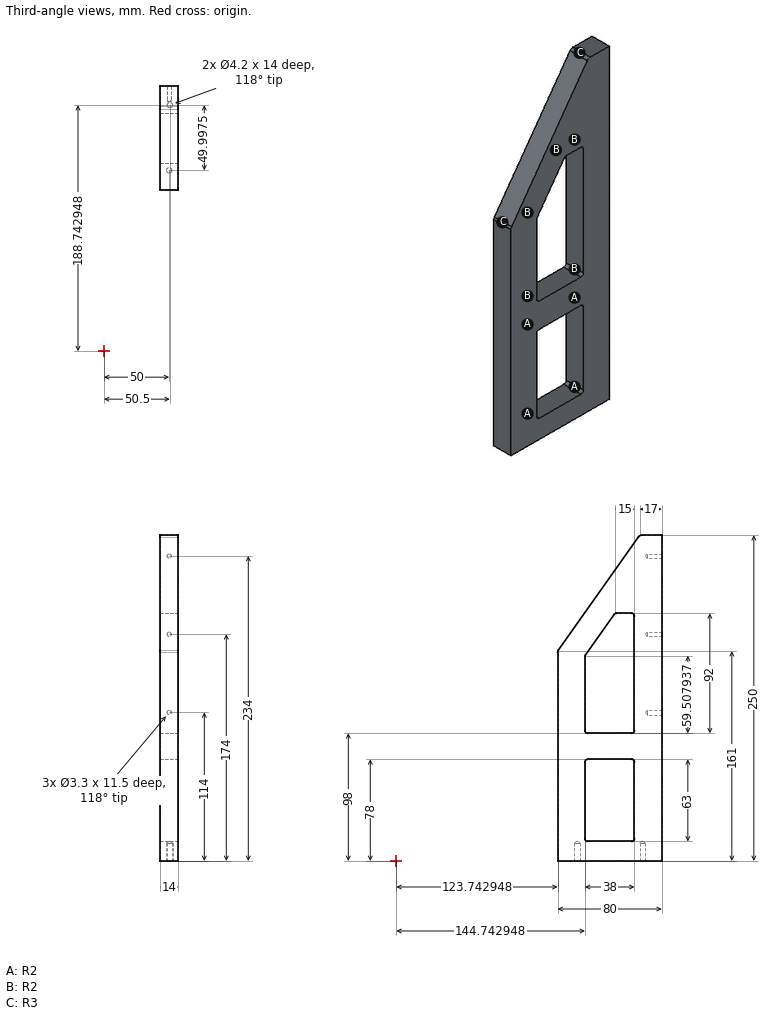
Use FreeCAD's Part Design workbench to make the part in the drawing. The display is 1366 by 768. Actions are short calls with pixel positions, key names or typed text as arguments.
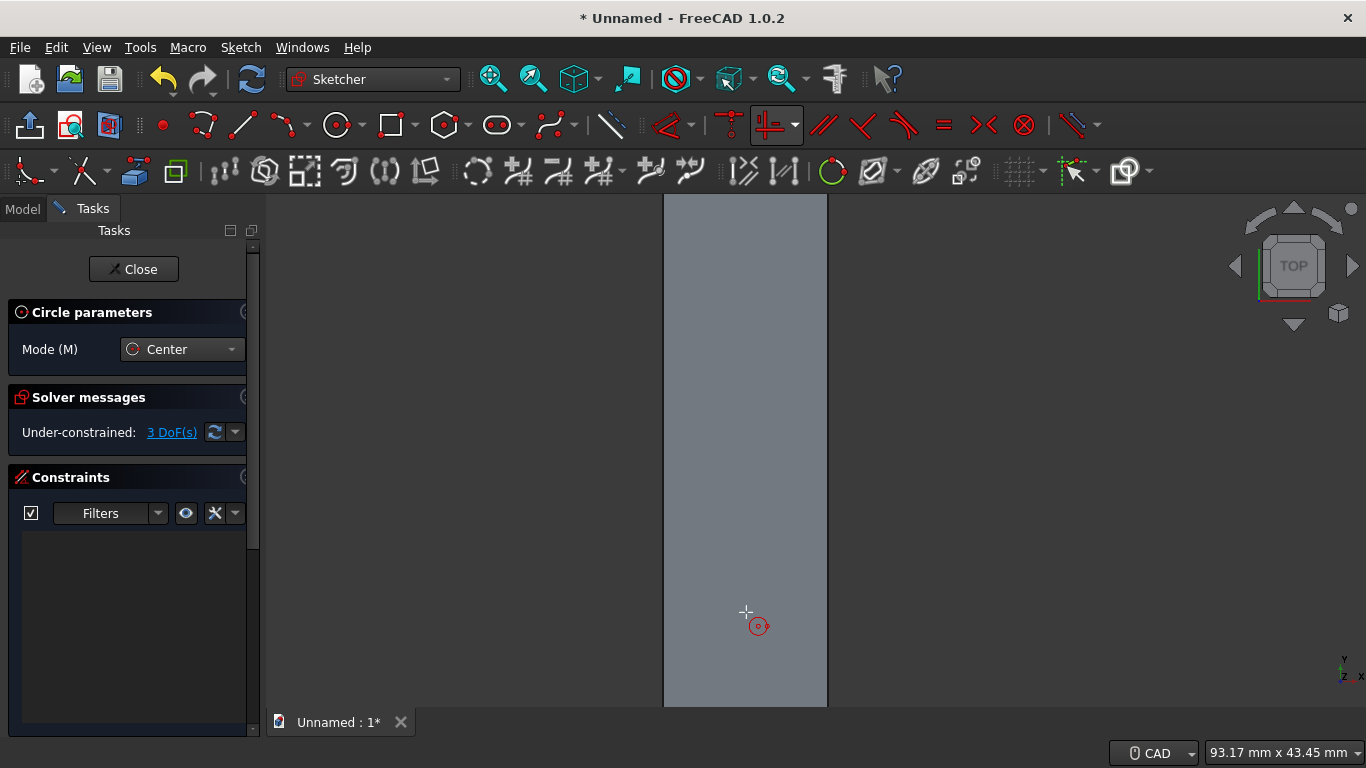
click(746, 612)
click(763, 595)
key(Escape)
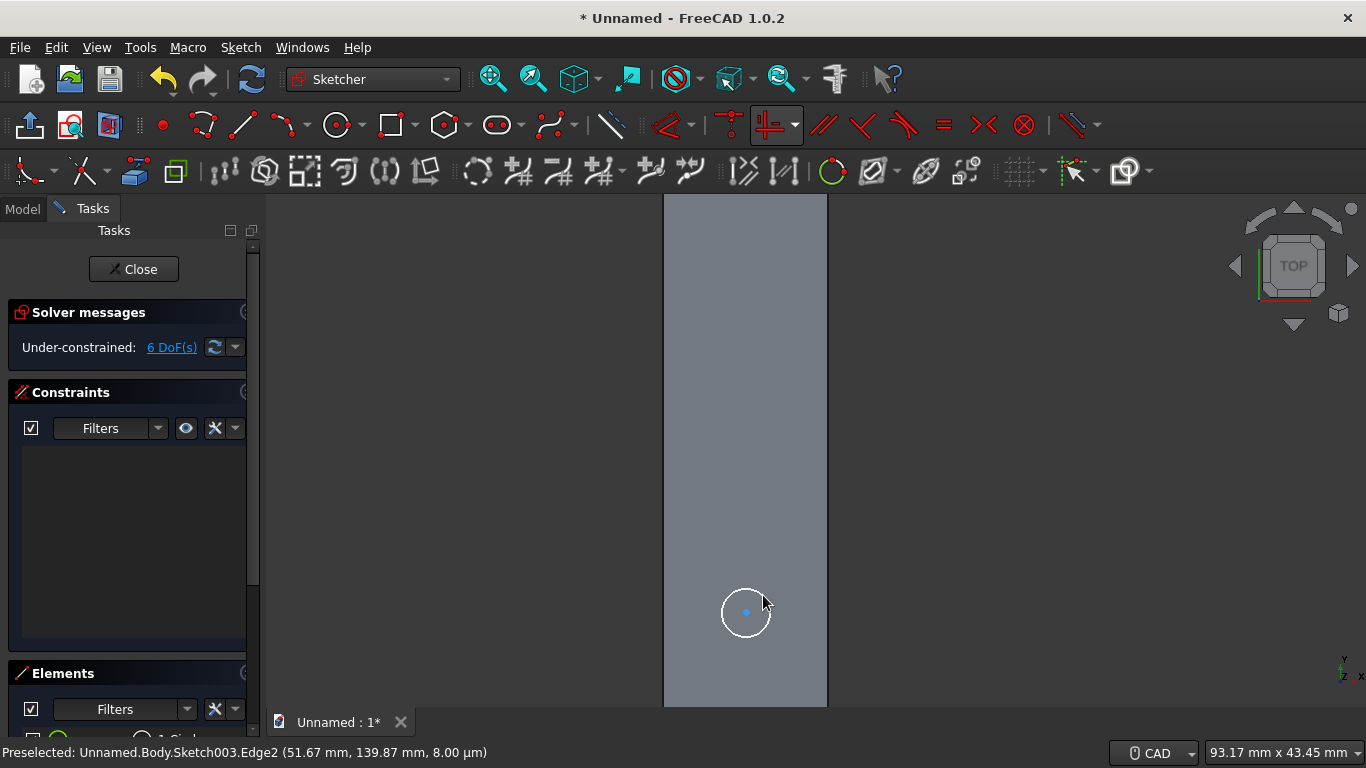
scroll(746, 613, down, 3)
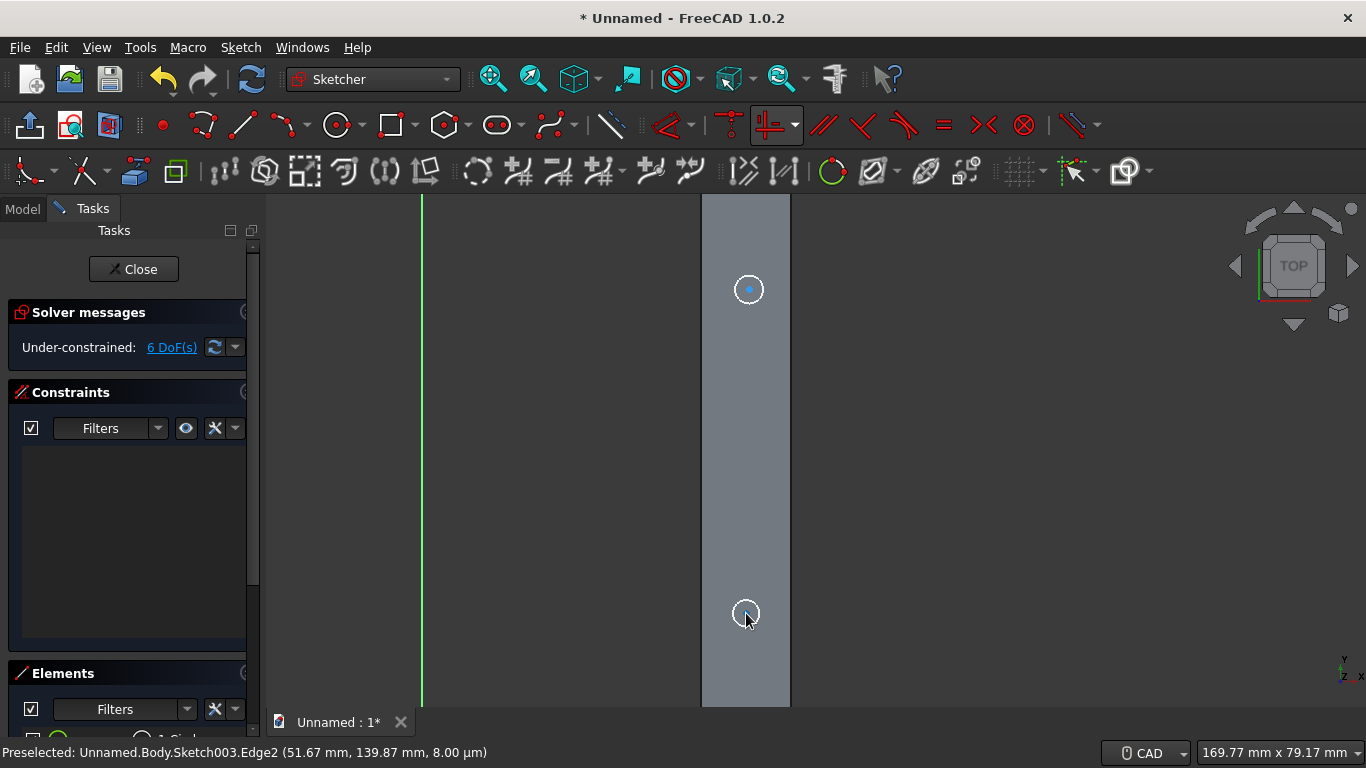
click(759, 280)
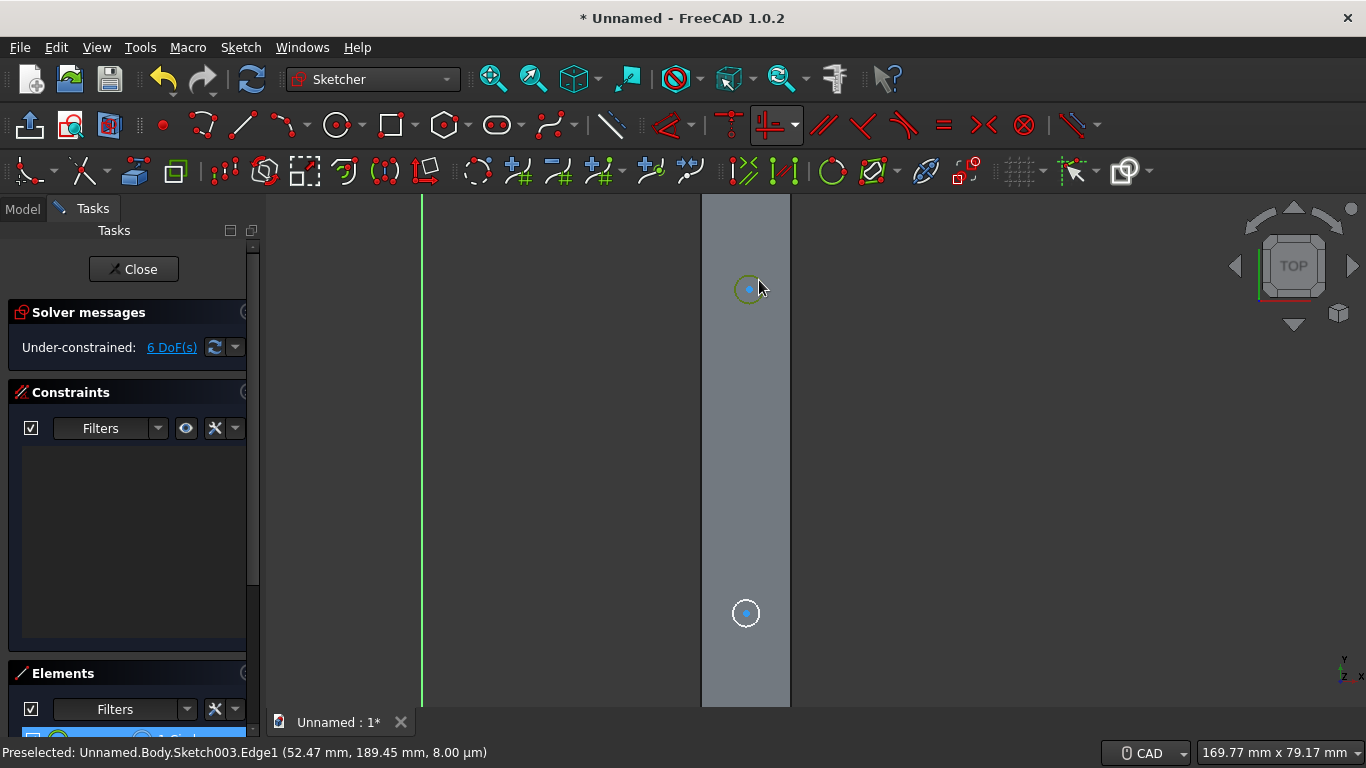
click(755, 604)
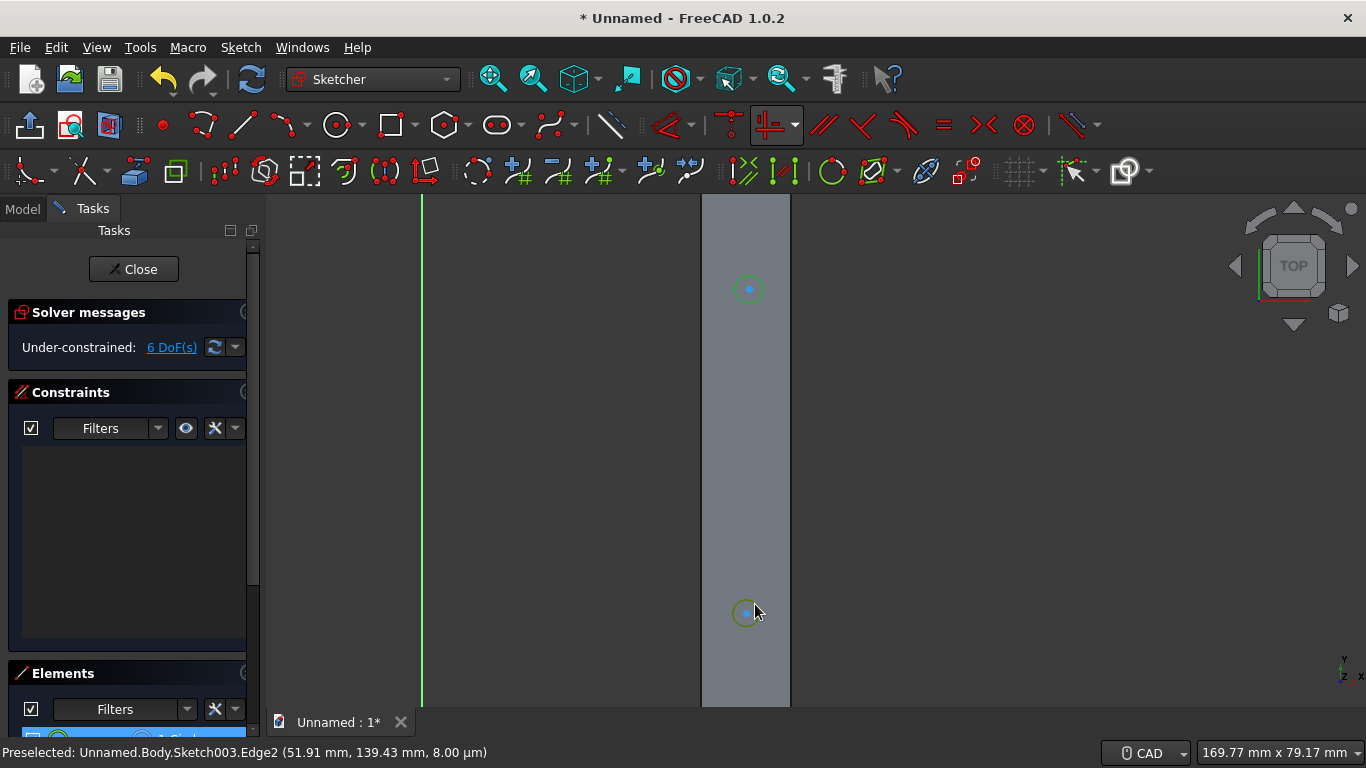
click(944, 126)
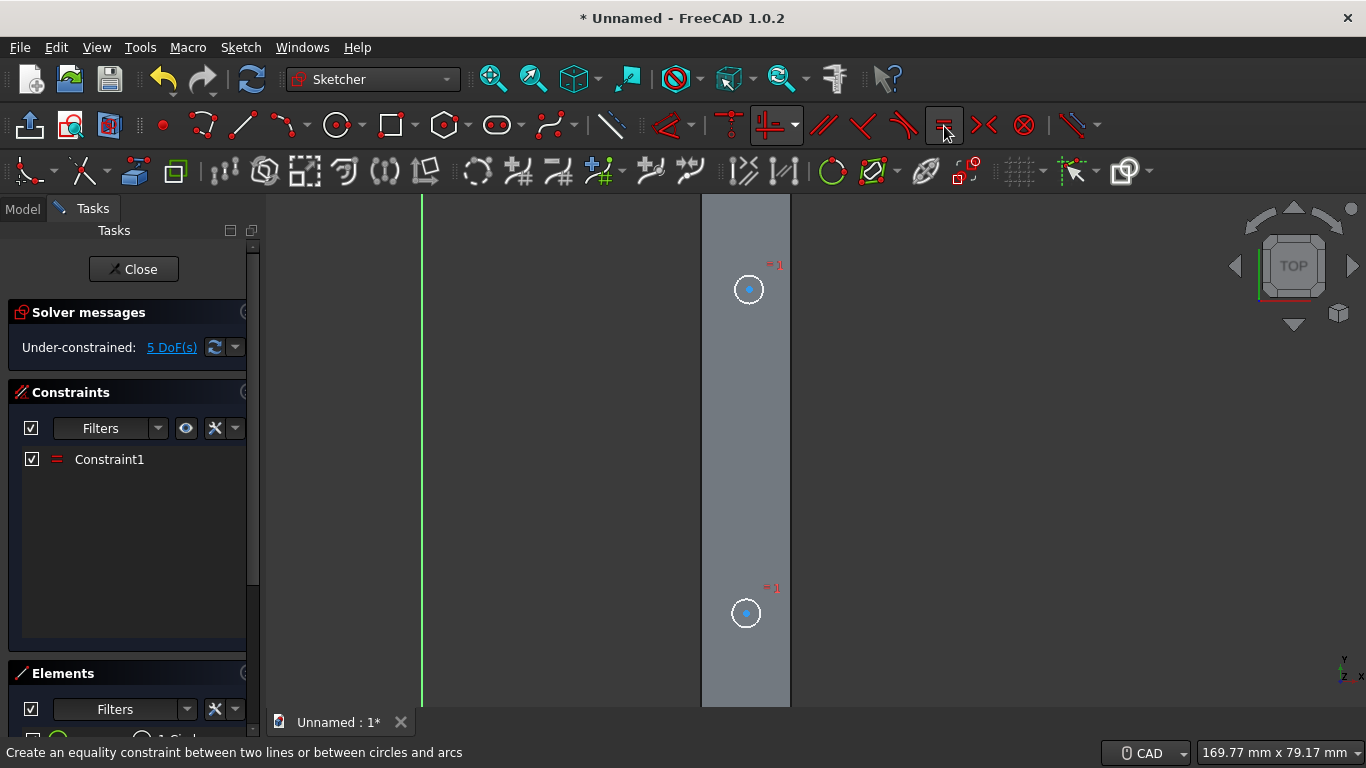
click(666, 126)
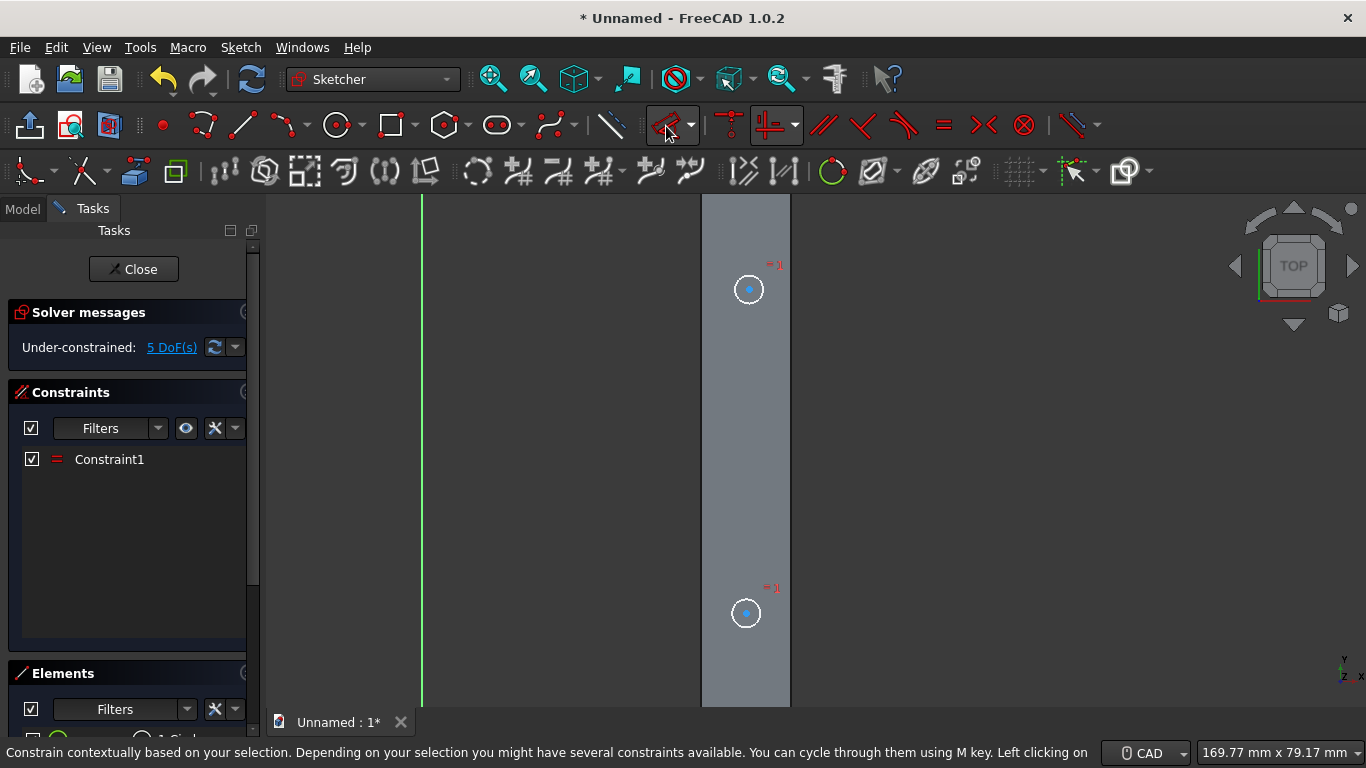
scroll(759, 280, up, 2)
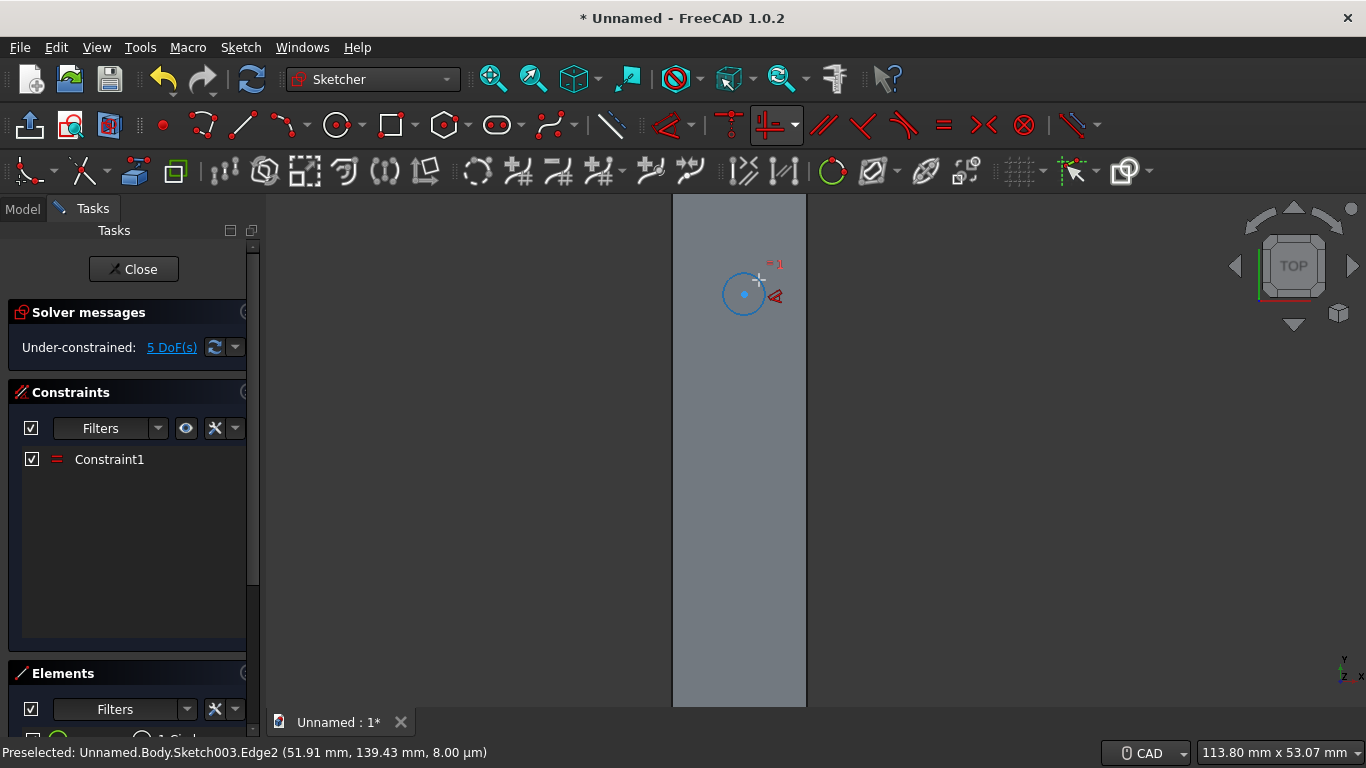
click(759, 279)
click(782, 256)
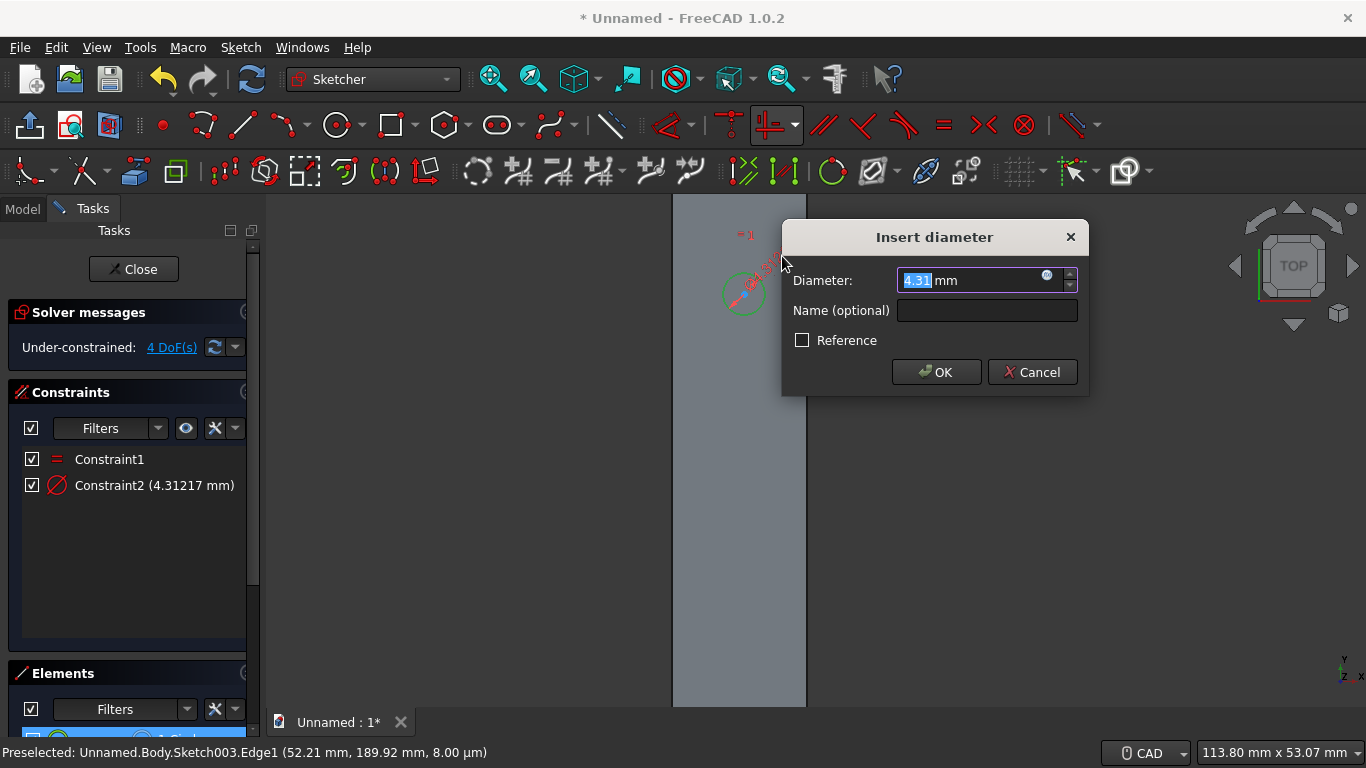
text(4.2)
key(Return)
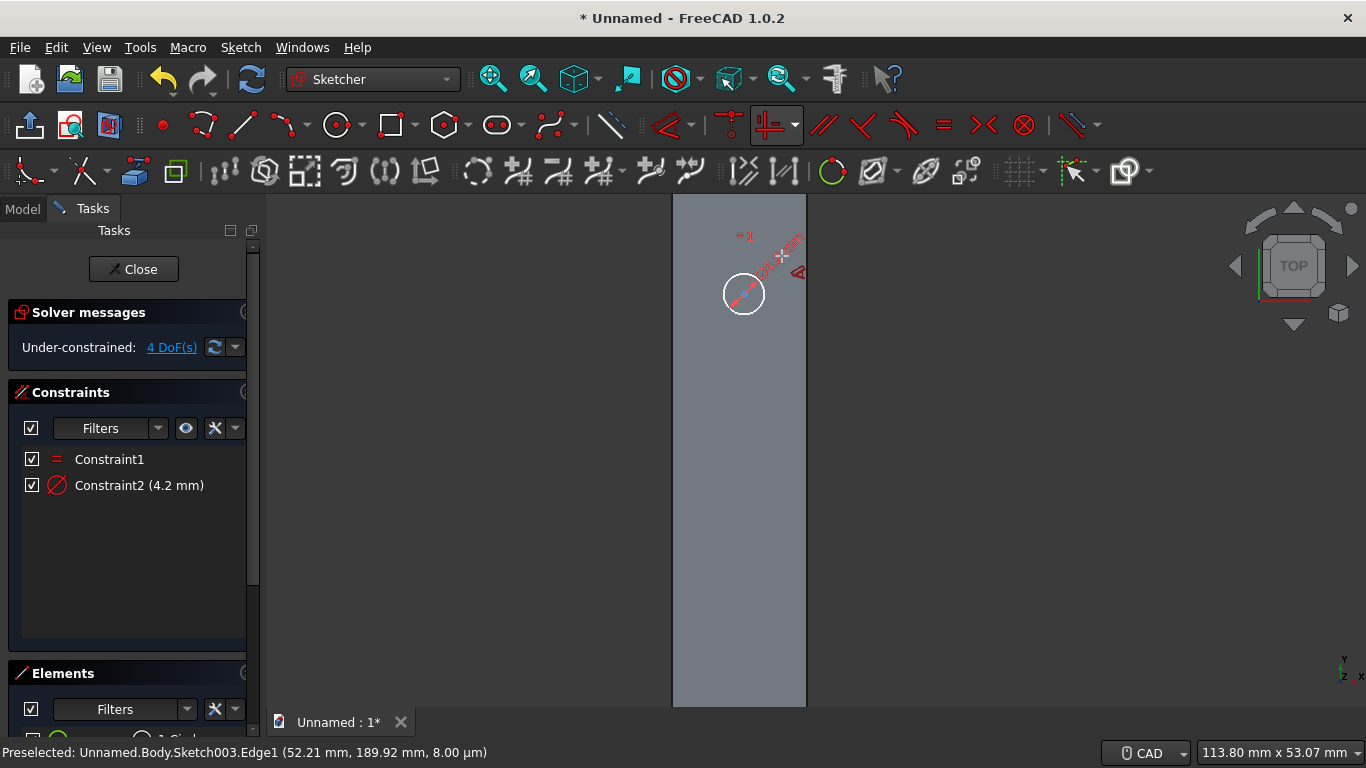
scroll(759, 279, down, 2)